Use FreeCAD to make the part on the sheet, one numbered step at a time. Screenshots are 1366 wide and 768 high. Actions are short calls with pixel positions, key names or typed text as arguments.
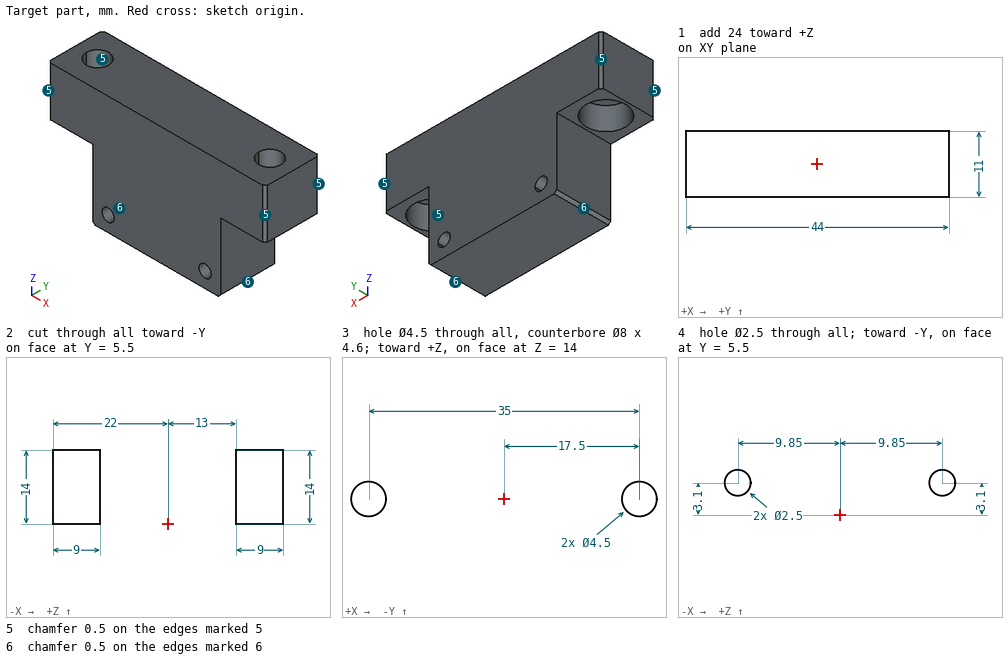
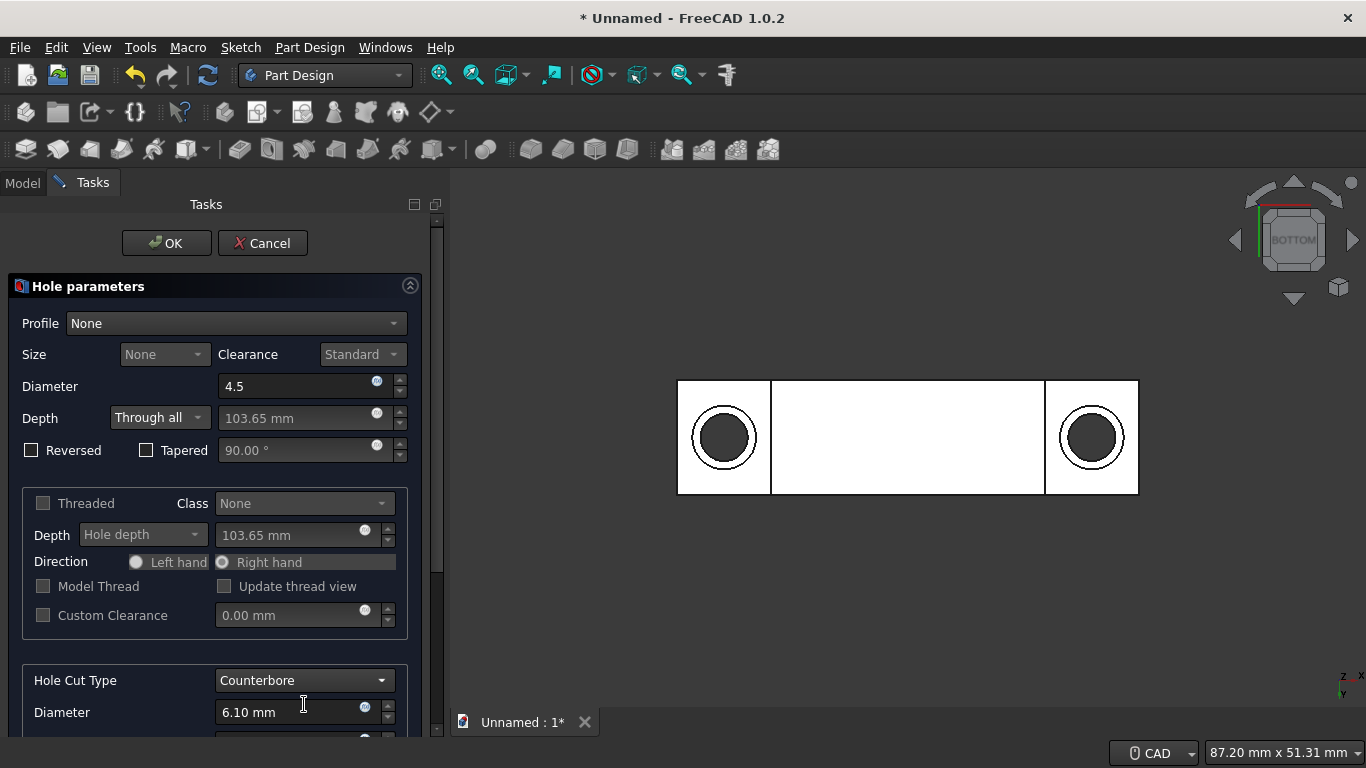
triple_click(298, 712)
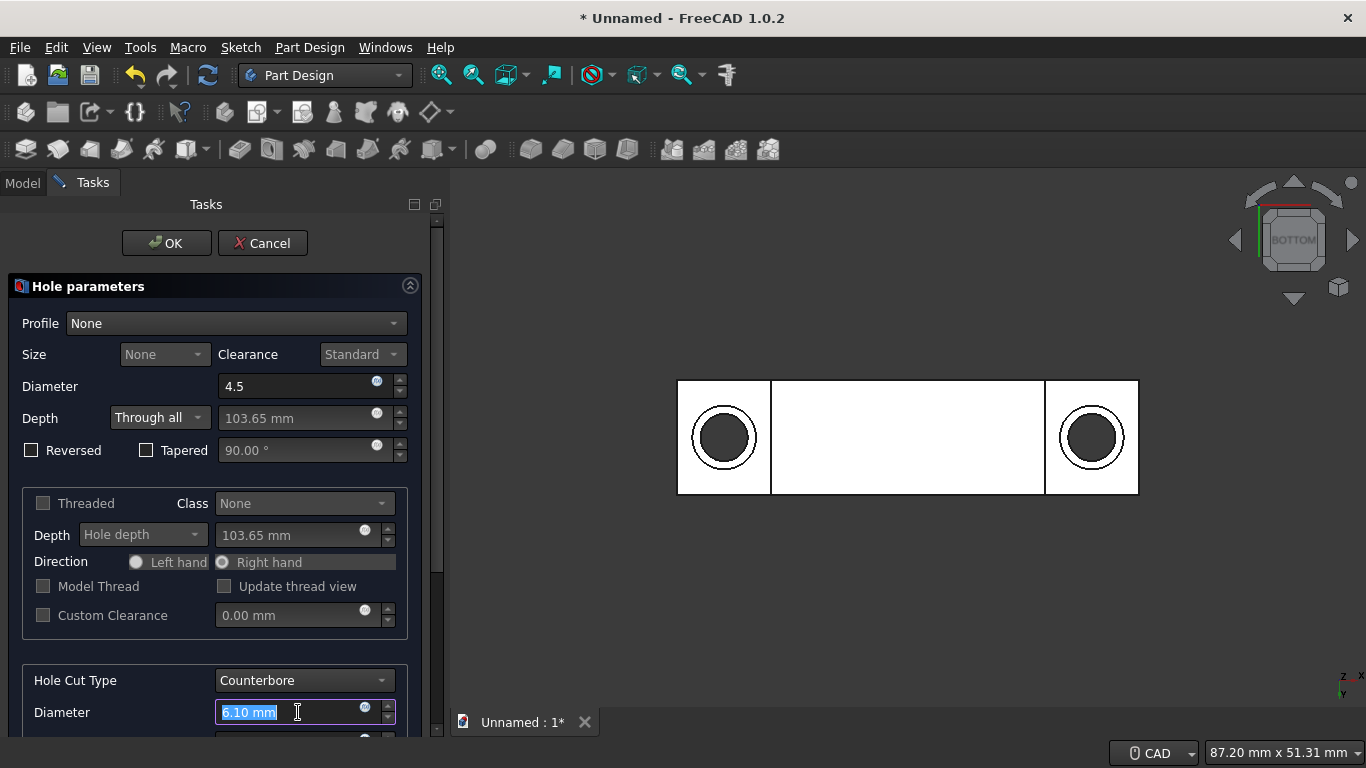
text(8)
key(Tab)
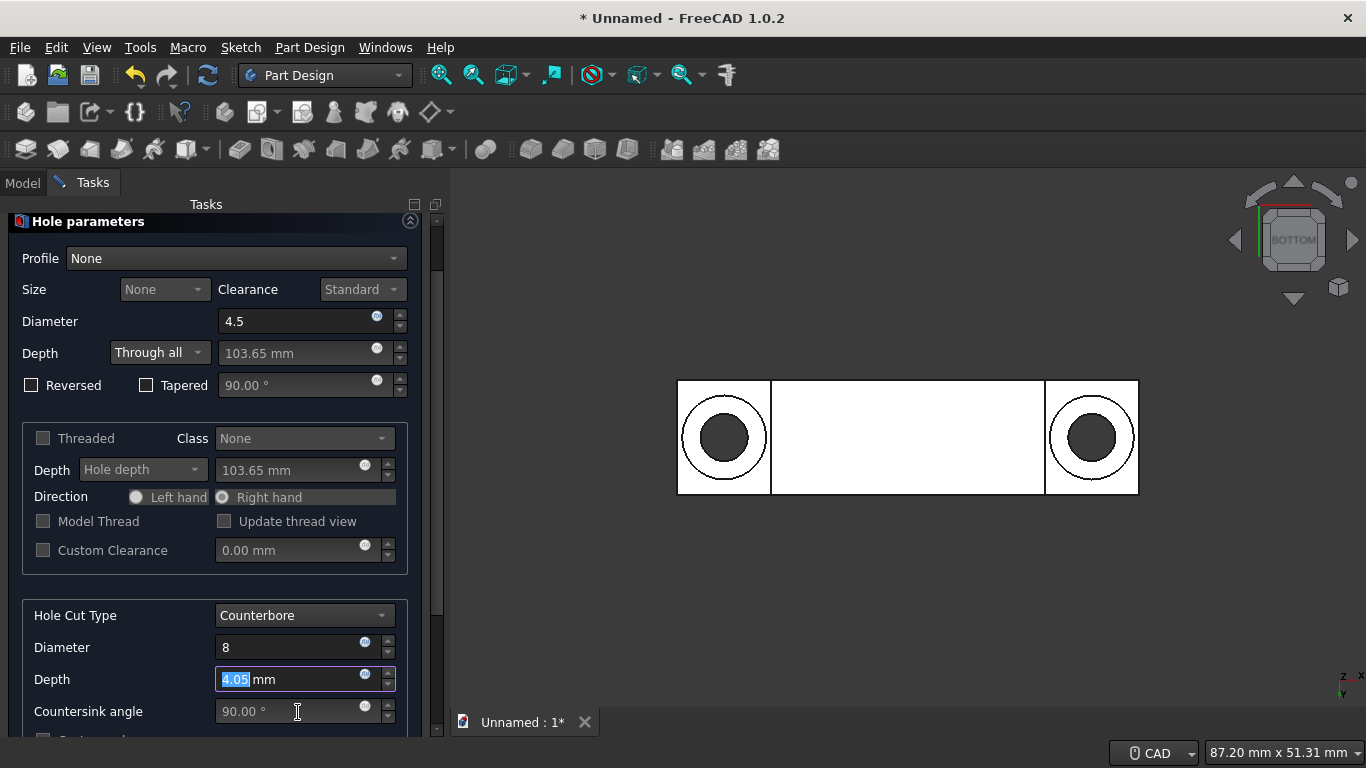
text(4.6)
key(Tab)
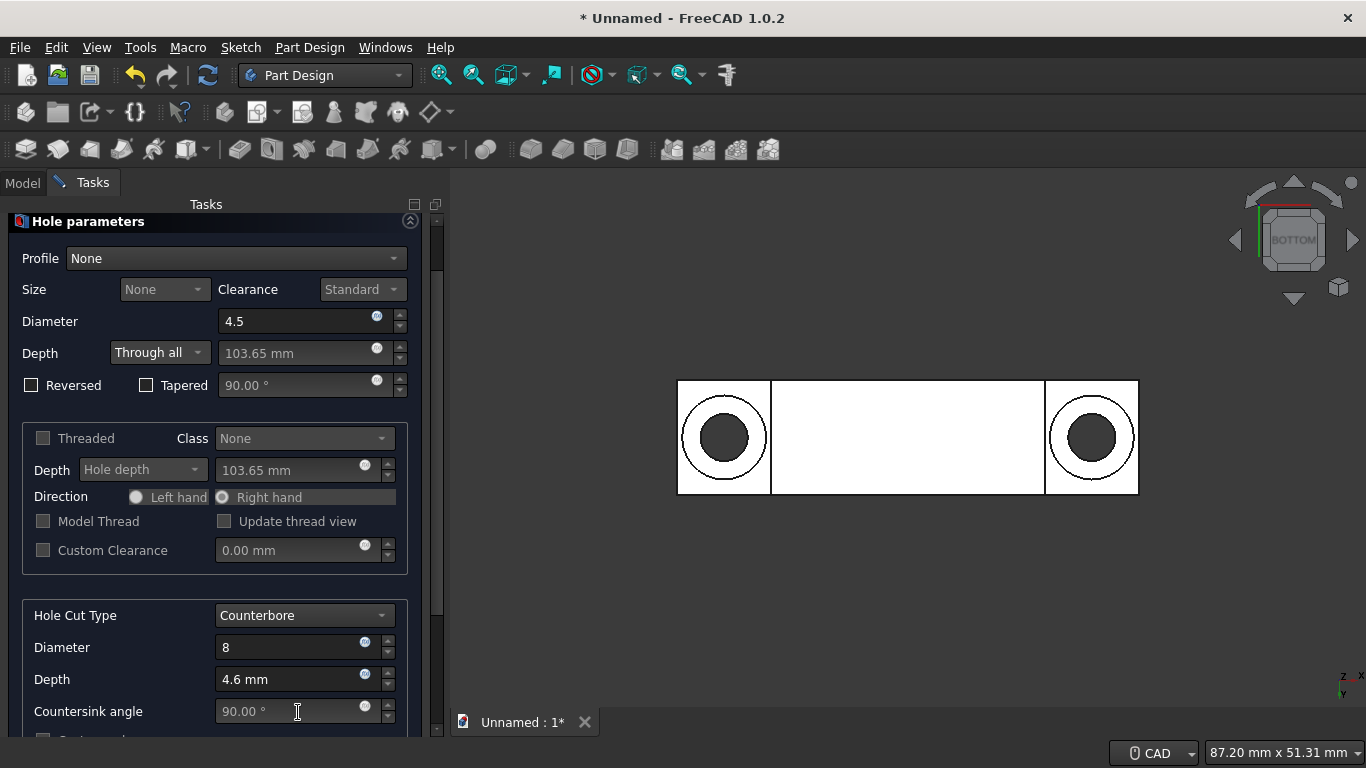
scroll(437, 475, up, 2)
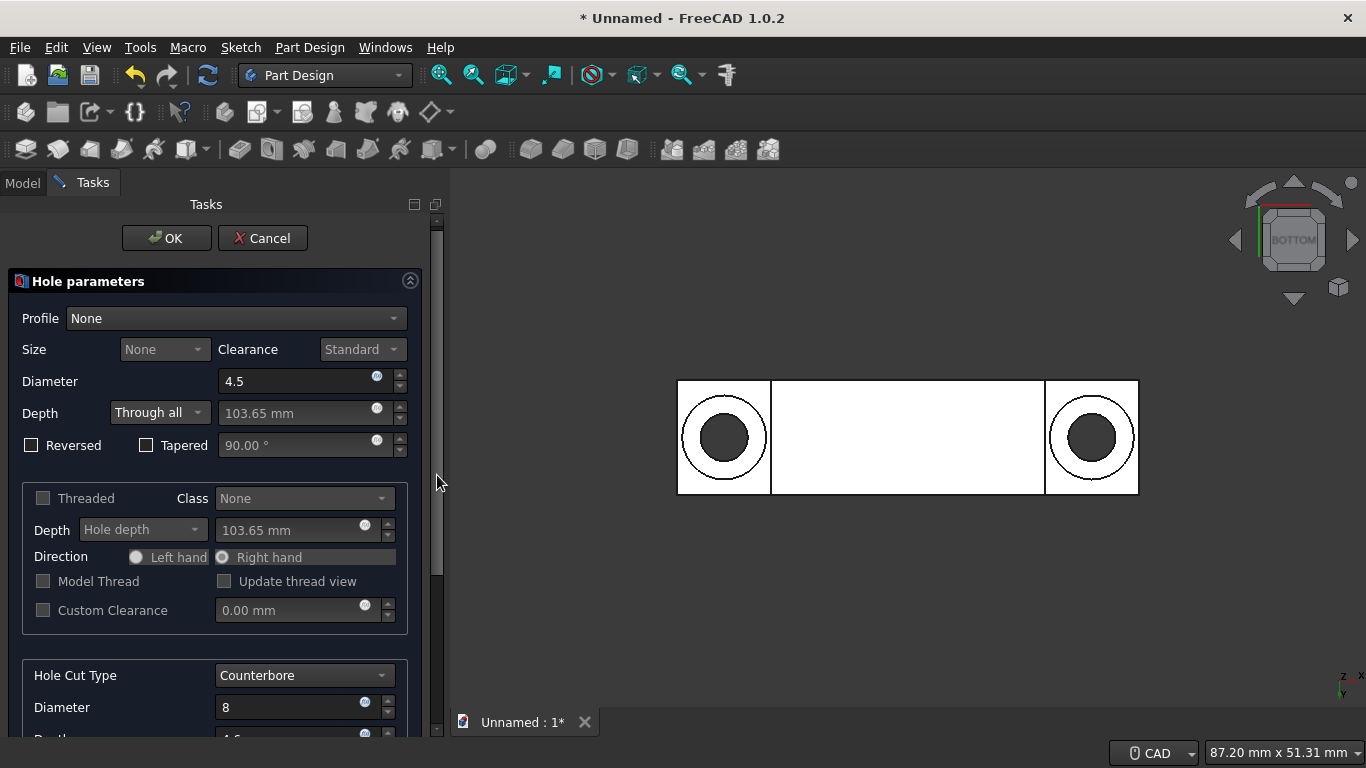
click(167, 243)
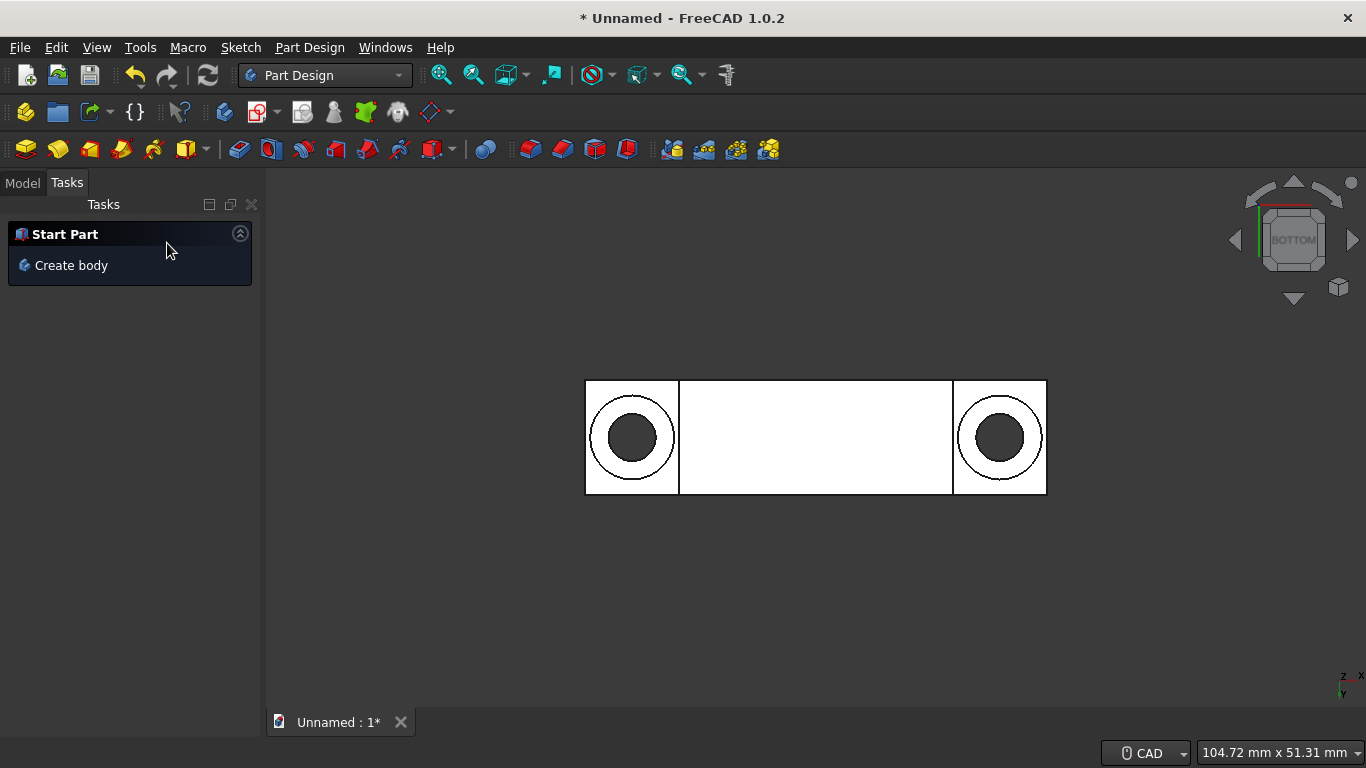
click(442, 76)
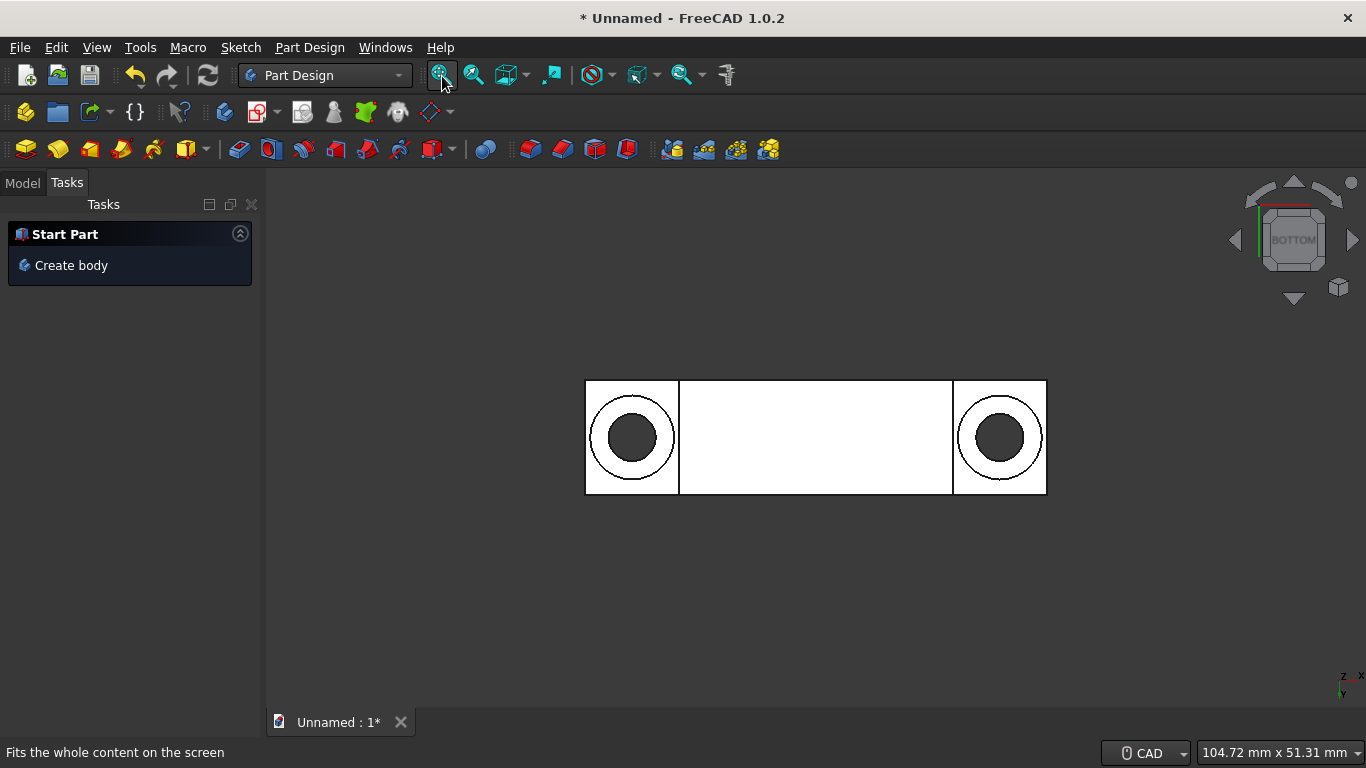
key(4)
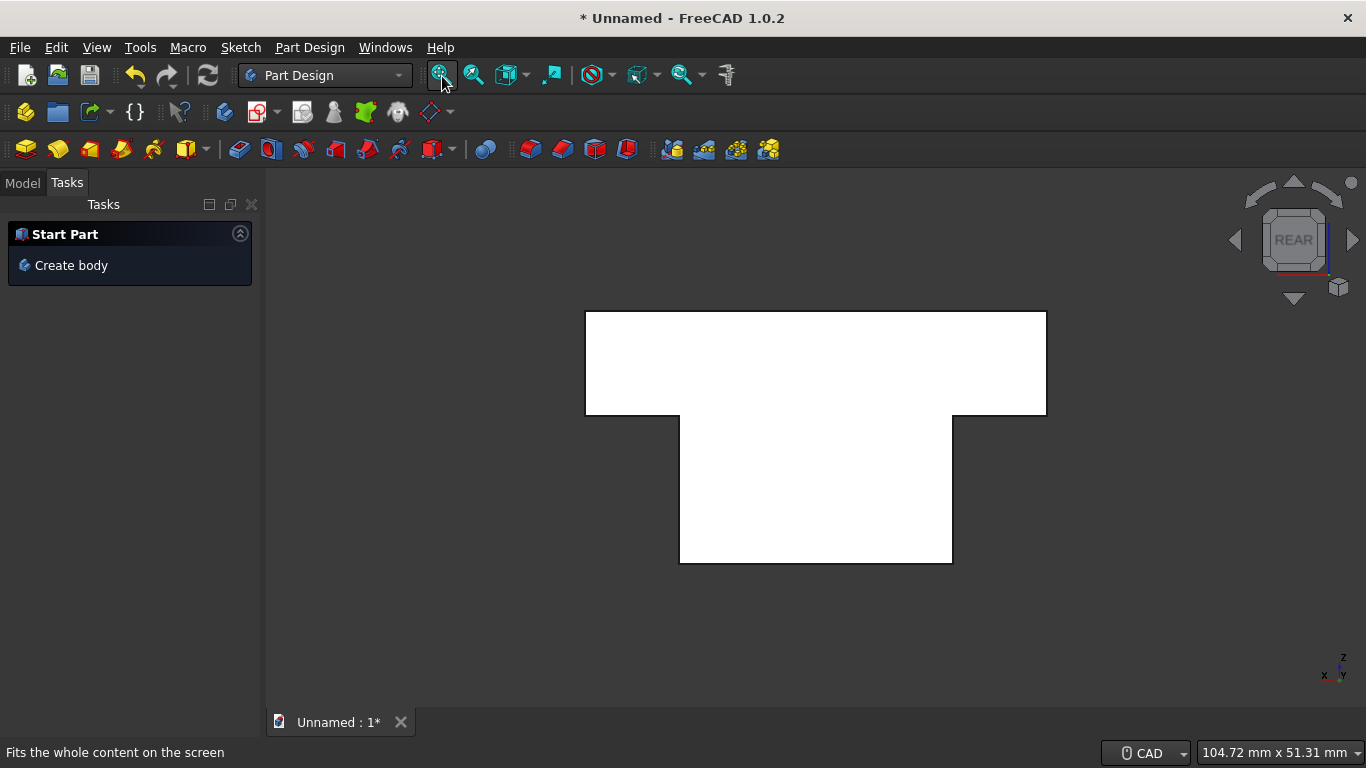
click(816, 437)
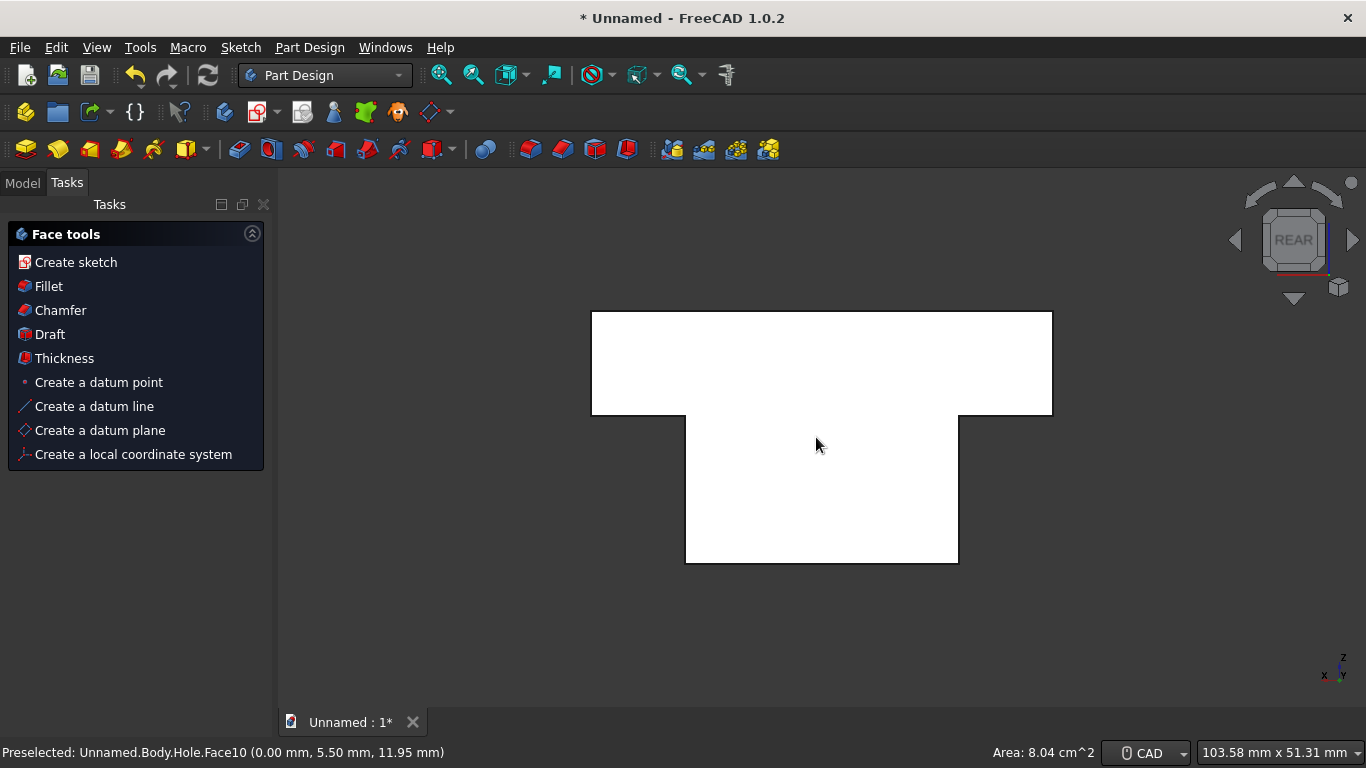
click(258, 112)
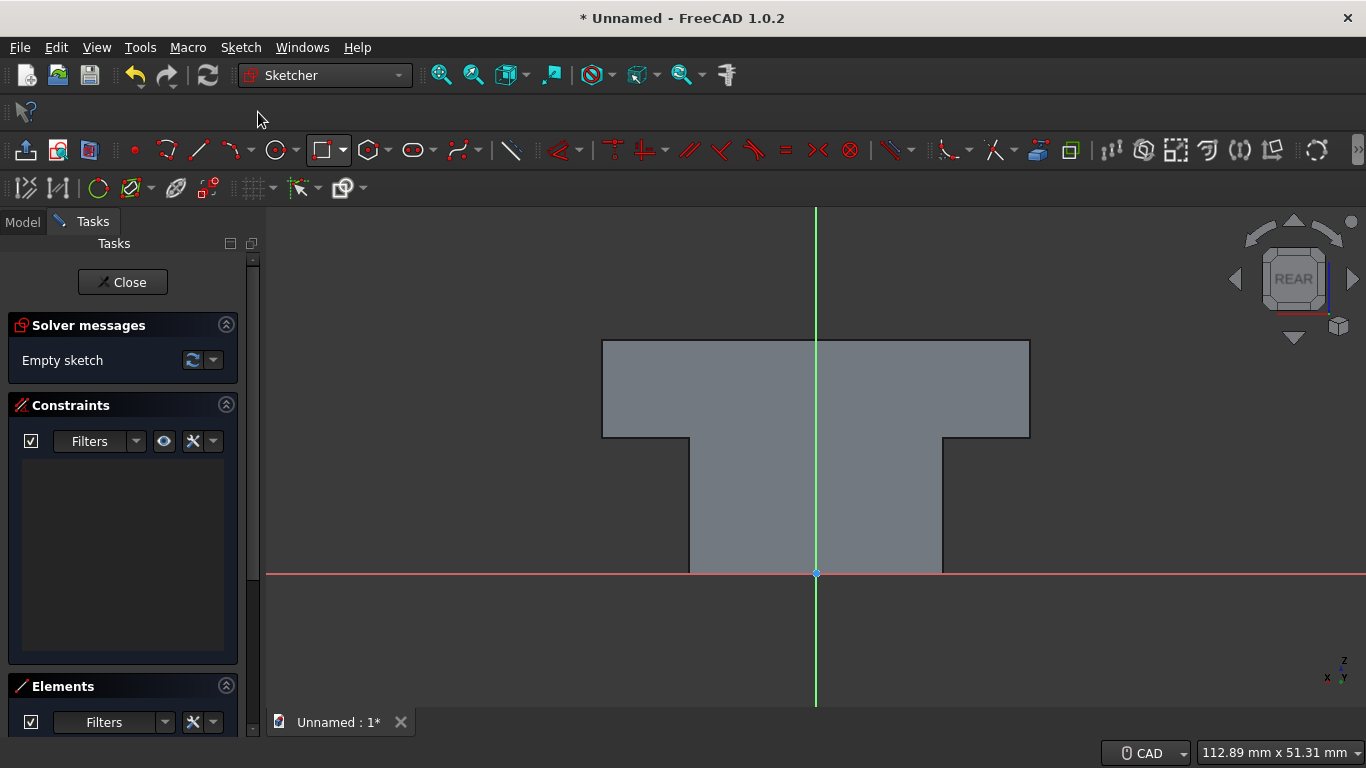
scroll(856, 608, up, 5)